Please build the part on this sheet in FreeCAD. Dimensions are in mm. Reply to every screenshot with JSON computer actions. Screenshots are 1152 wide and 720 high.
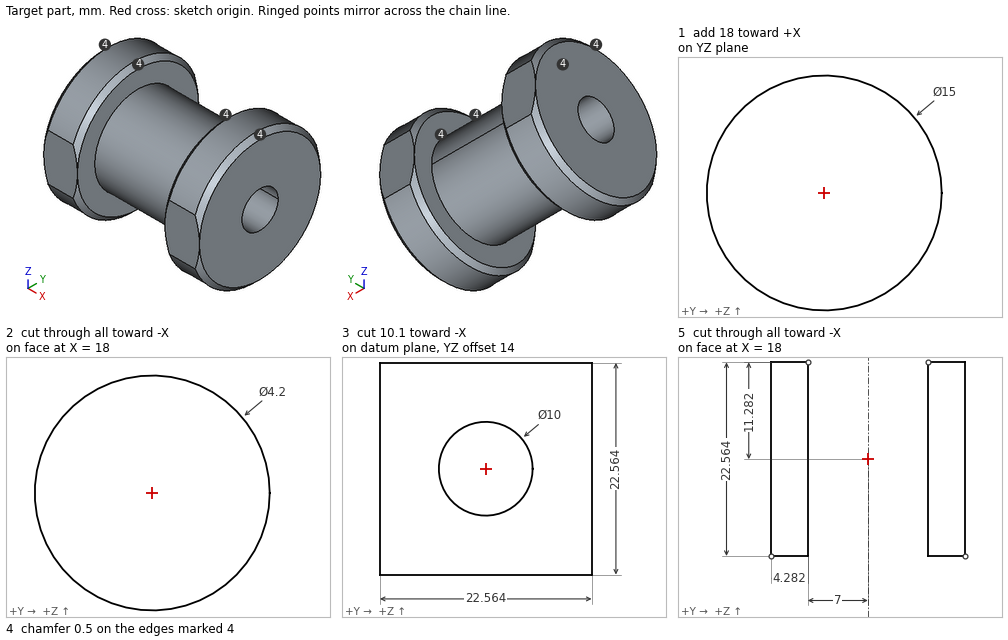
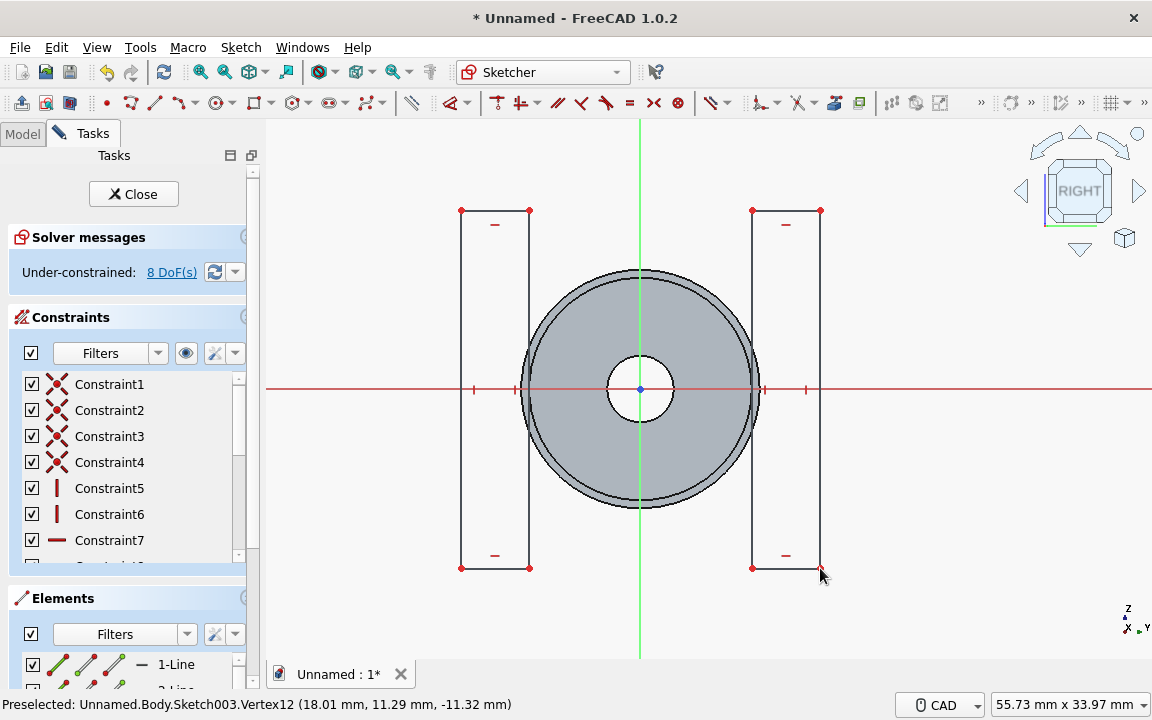
{"action": "left_click", "coordinate": [529, 211]}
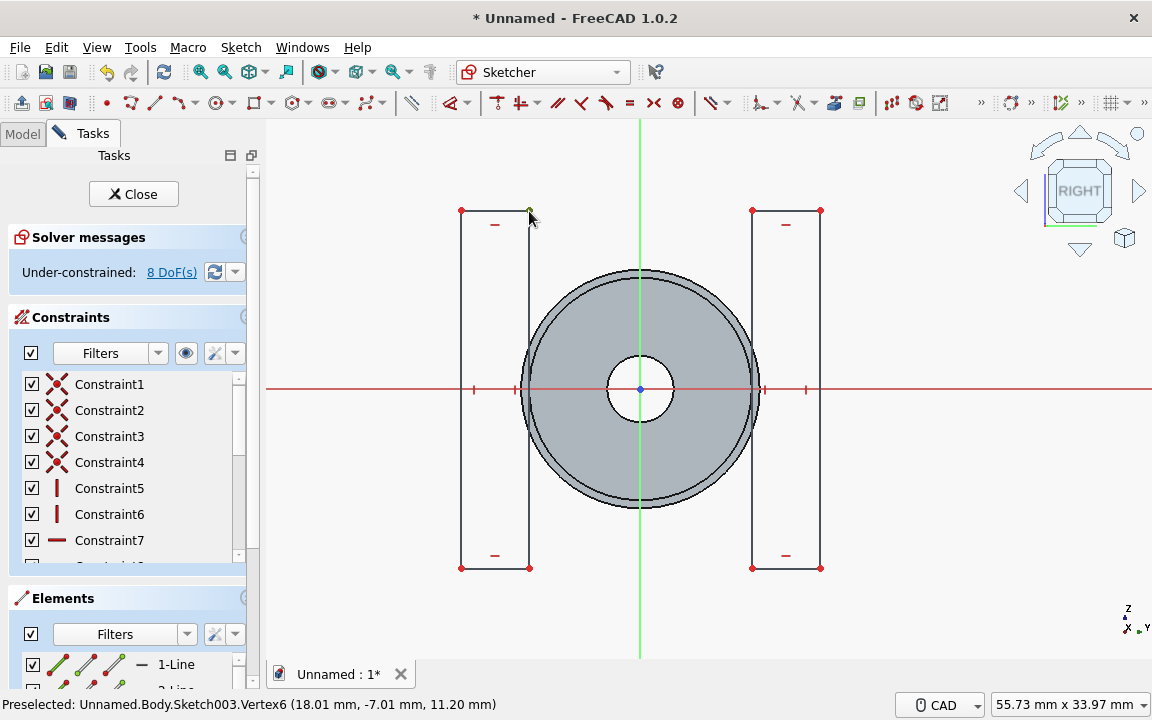
{"action": "left_click", "coordinate": [752, 211]}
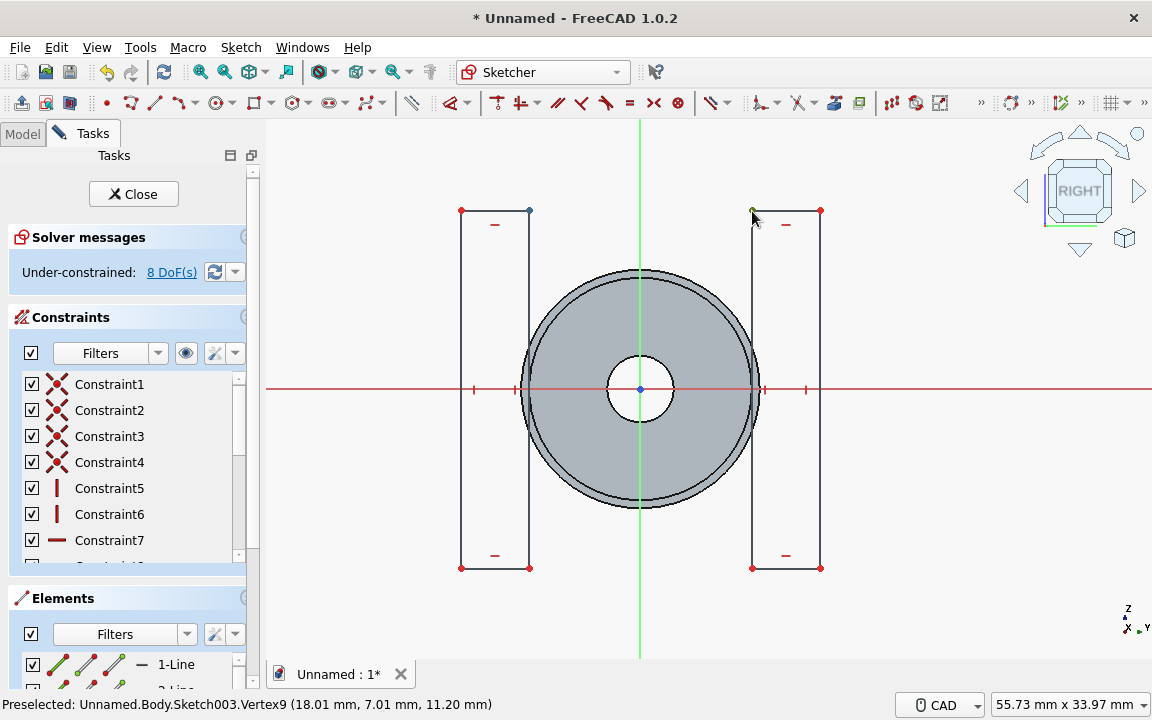
{"action": "left_click", "coordinate": [640, 596]}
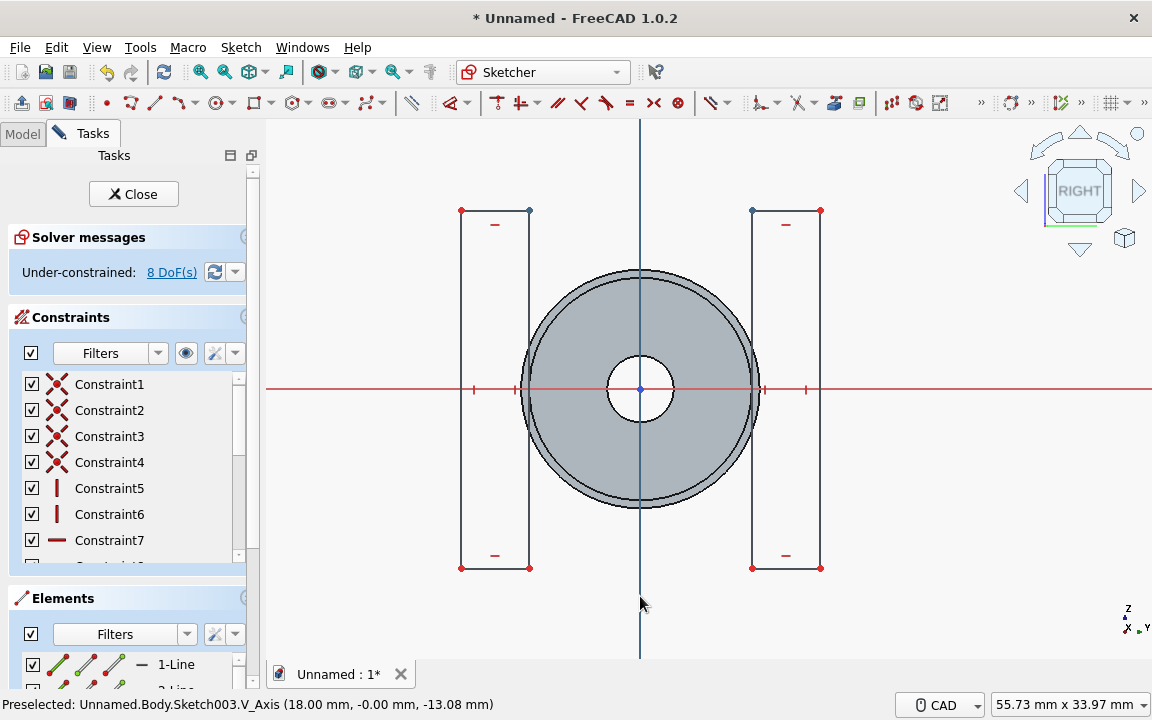
{"action": "left_click", "coordinate": [654, 104]}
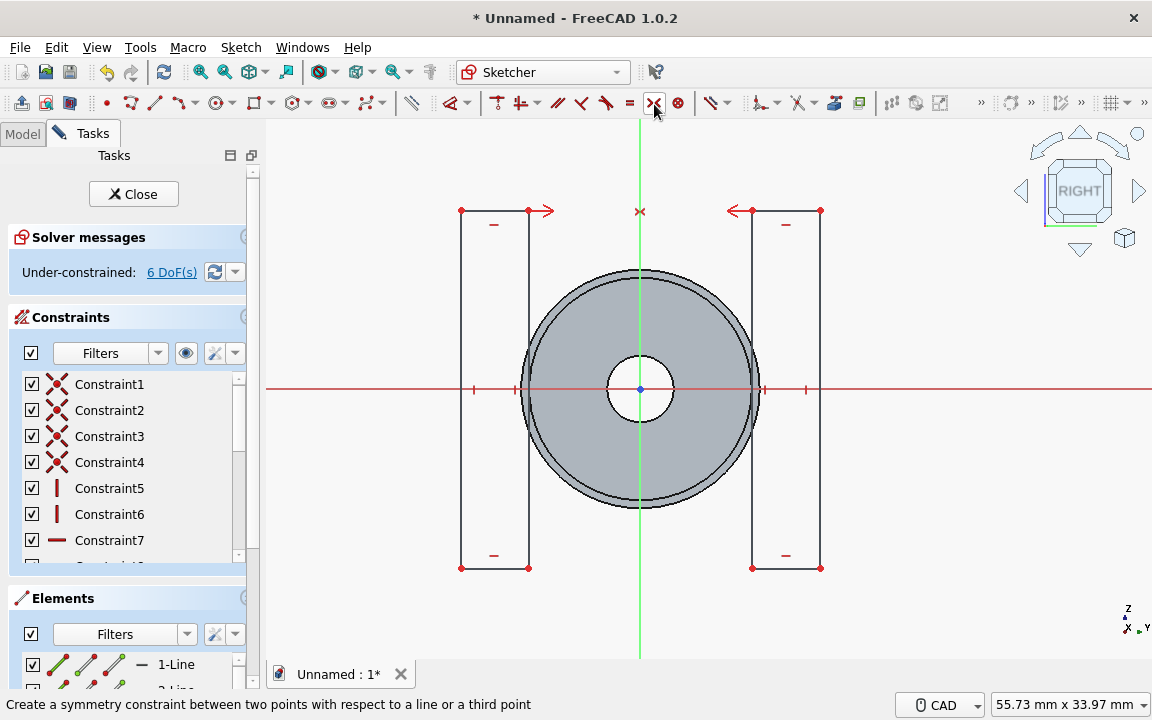
{"action": "left_click", "coordinate": [461, 569]}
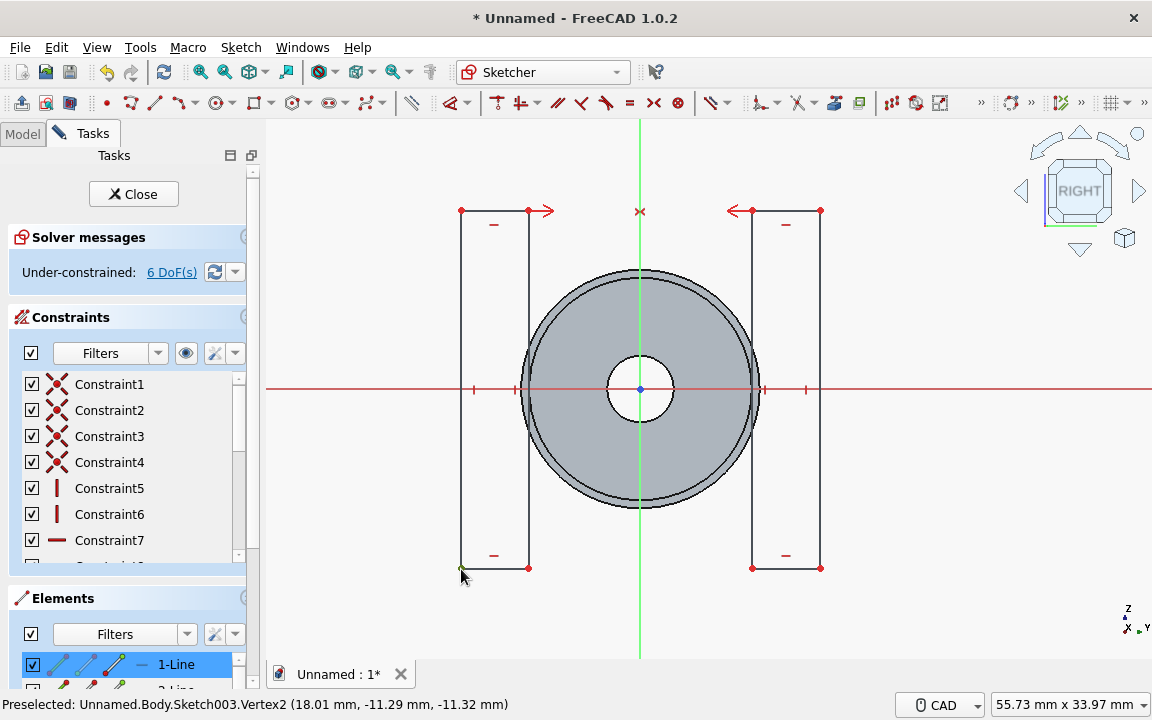
{"action": "left_click", "coordinate": [820, 569]}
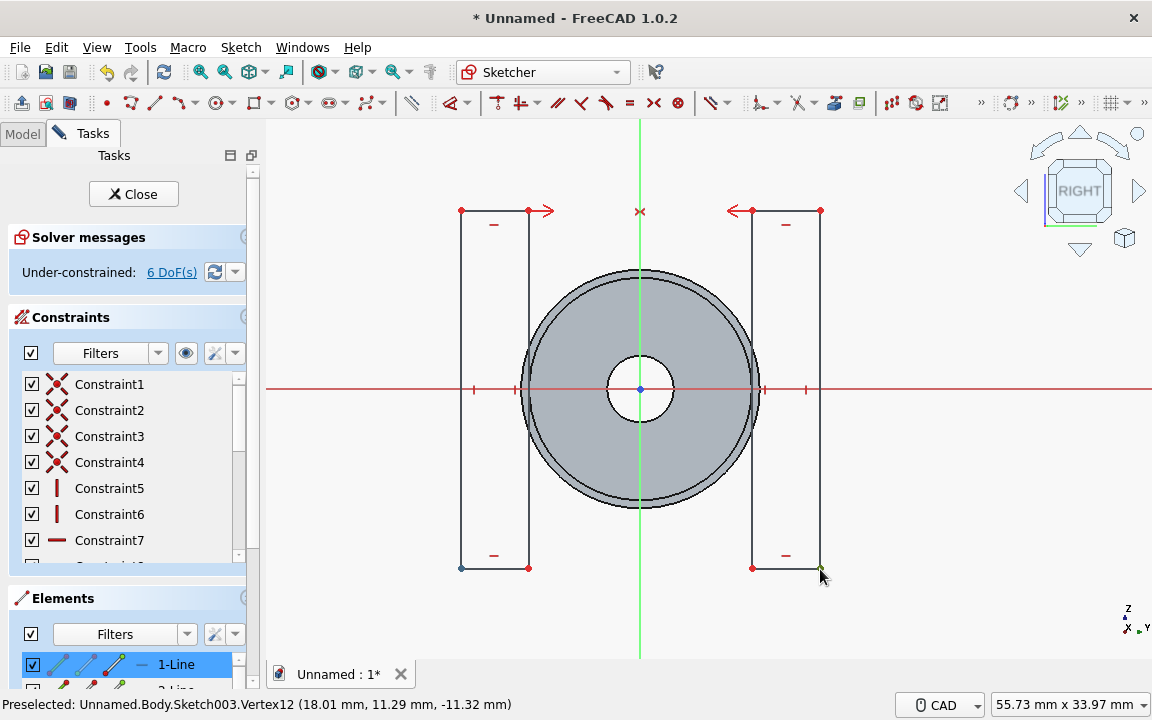
{"action": "left_click", "coordinate": [640, 596]}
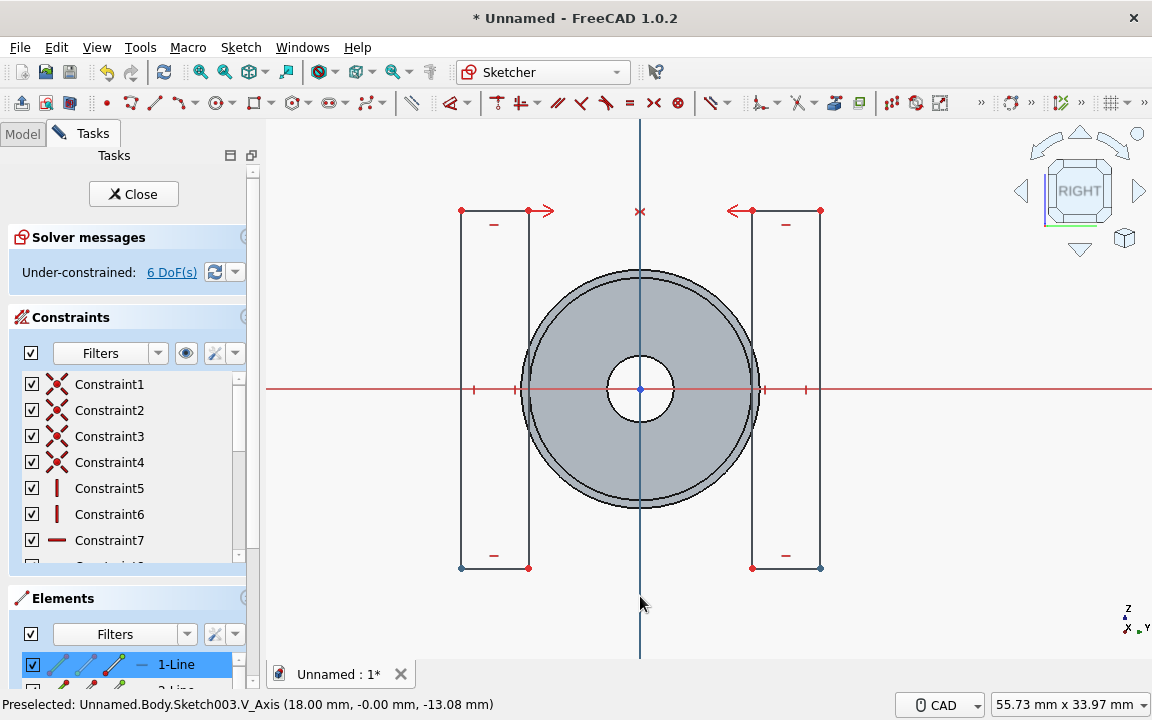
{"action": "left_click", "coordinate": [654, 104]}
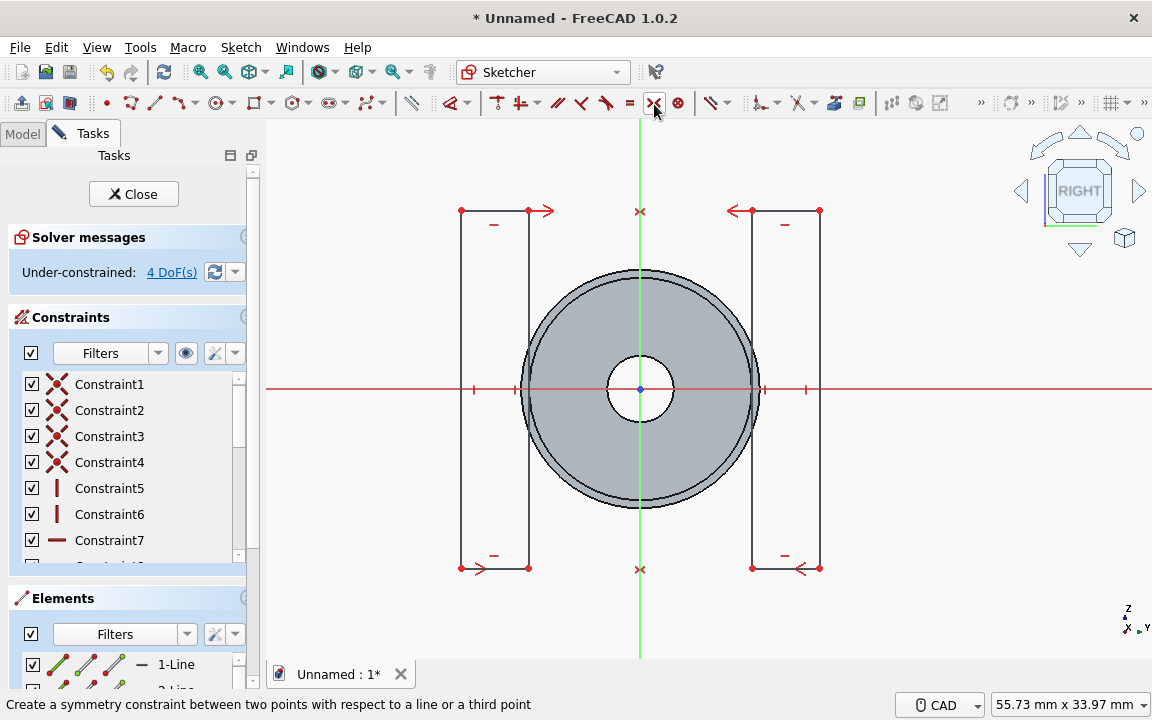
{"action": "left_click", "coordinate": [450, 104]}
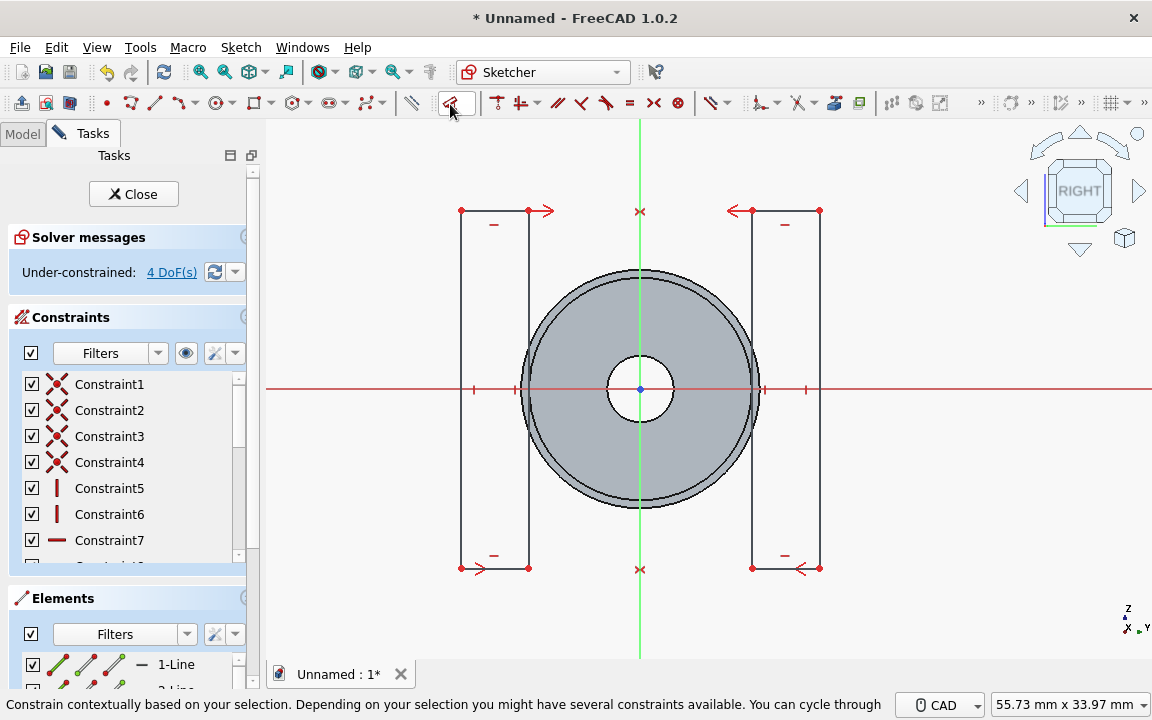
{"action": "left_click", "coordinate": [529, 569]}
{"action": "left_click", "coordinate": [585, 603]}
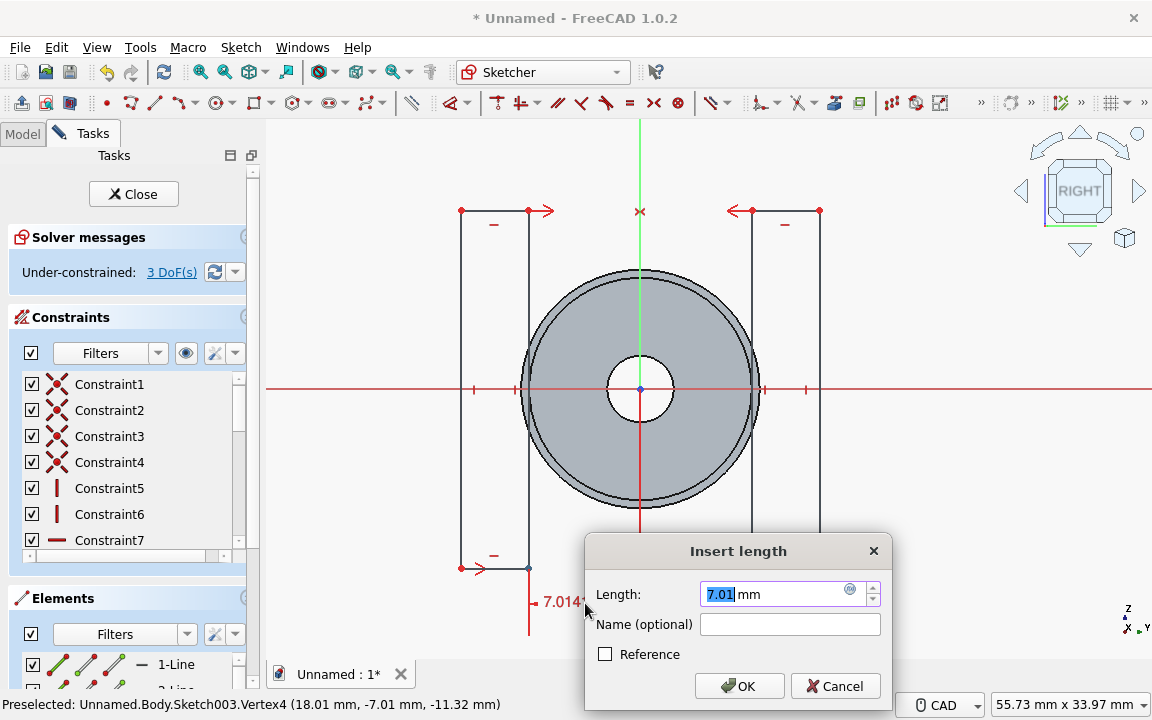
{"action": "type", "text": "7"}
{"action": "key", "text": "Return"}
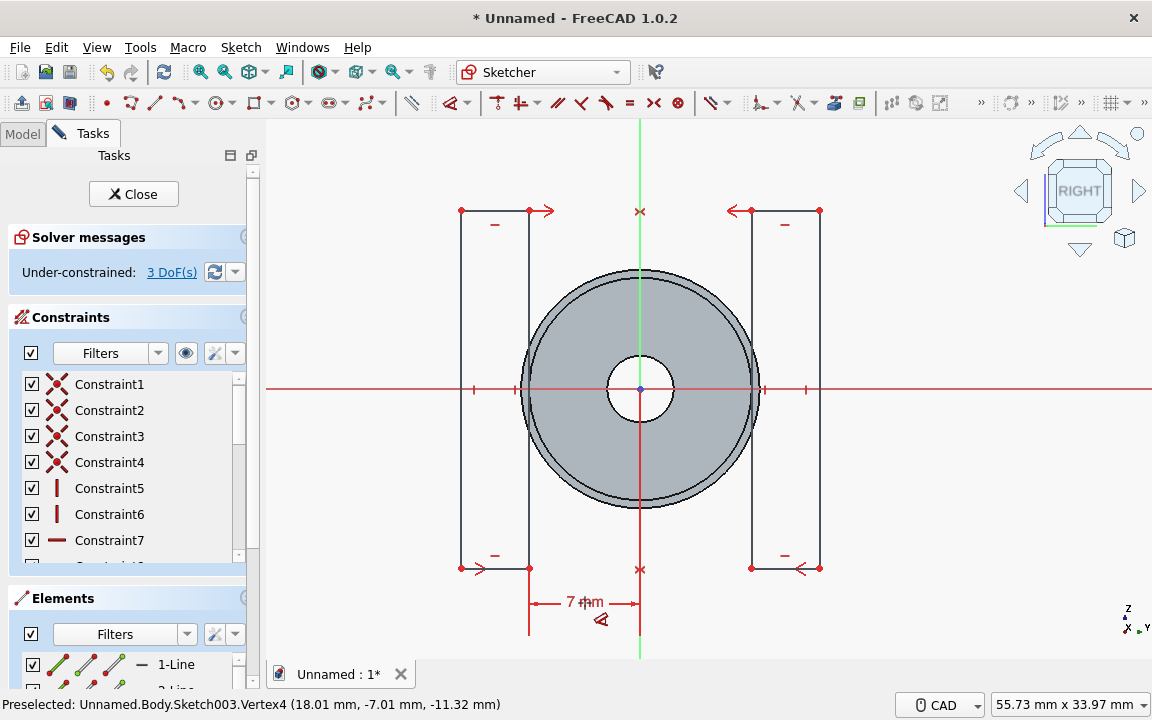
{"action": "left_click", "coordinate": [481, 569]}
{"action": "left_click", "coordinate": [495, 603]}